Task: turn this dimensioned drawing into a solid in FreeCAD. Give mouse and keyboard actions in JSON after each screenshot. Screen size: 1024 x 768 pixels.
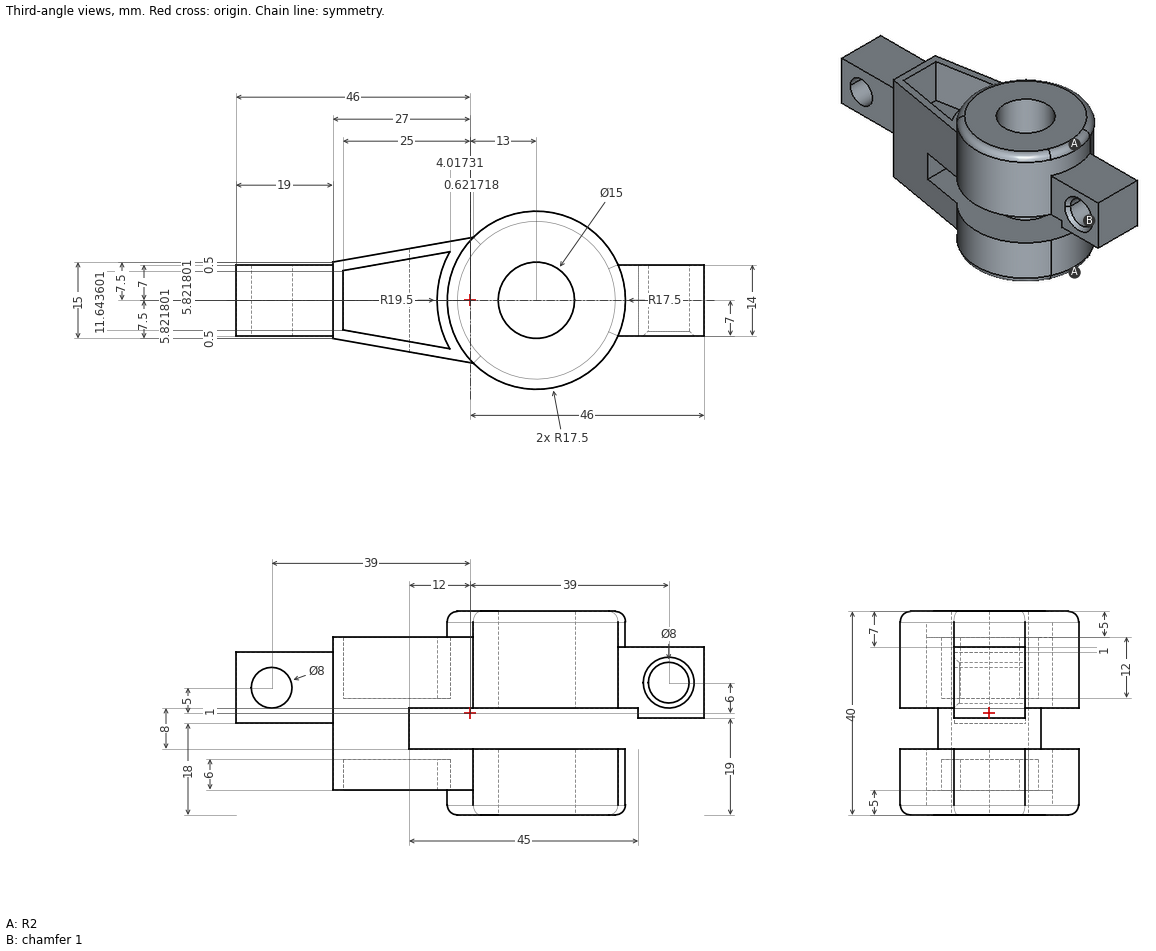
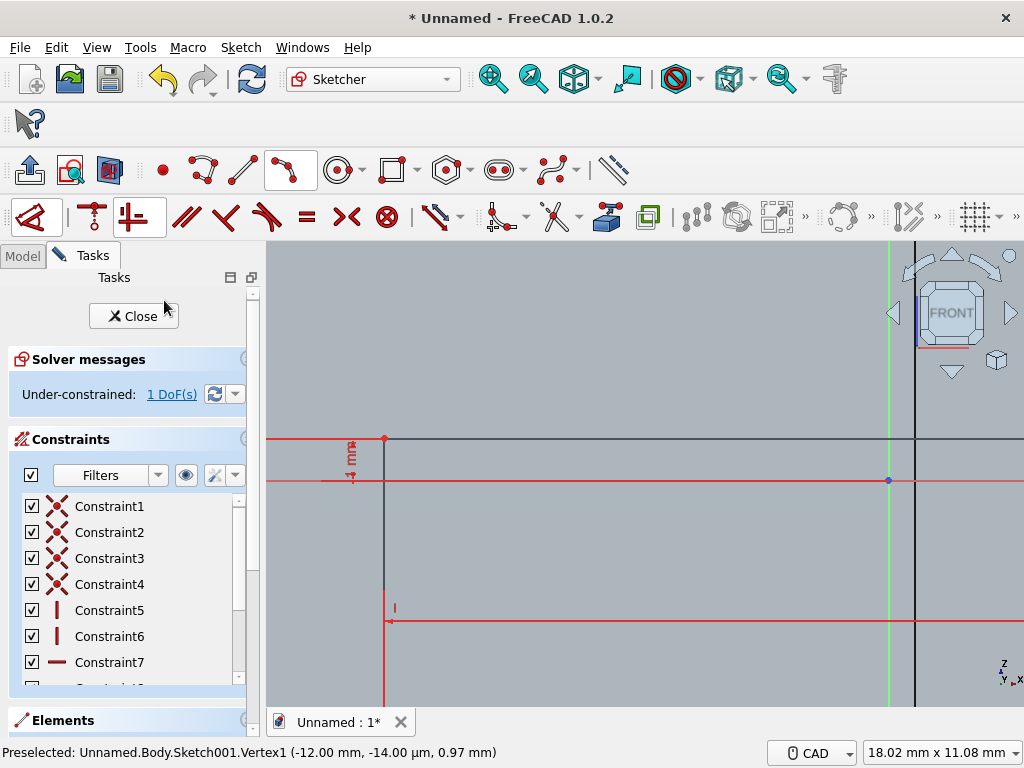
{"action": "scroll", "coordinate": [386, 440], "scroll_direction": "down", "scroll_amount": 8}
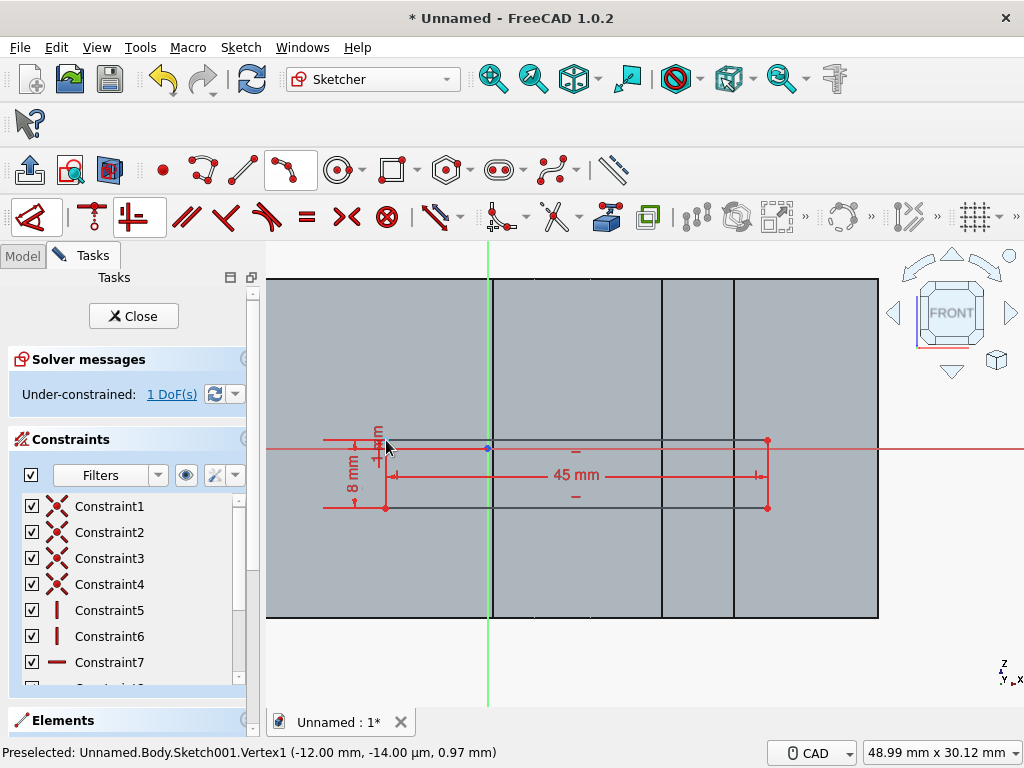
{"action": "left_click", "coordinate": [386, 440]}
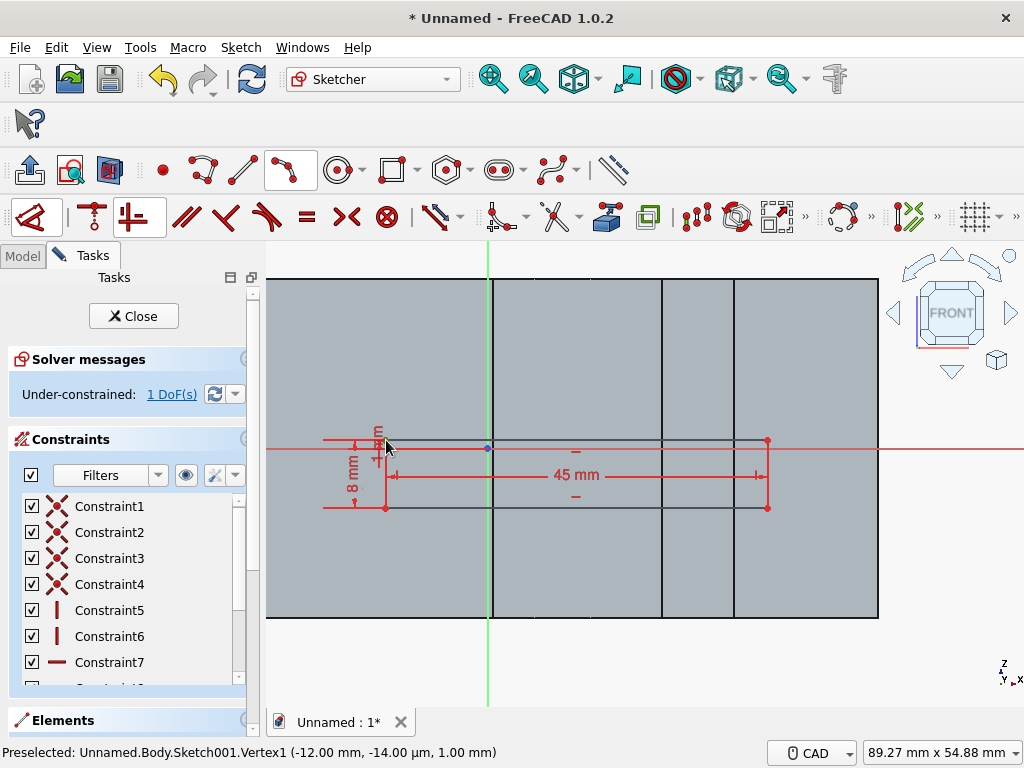
{"action": "key", "text": "l"}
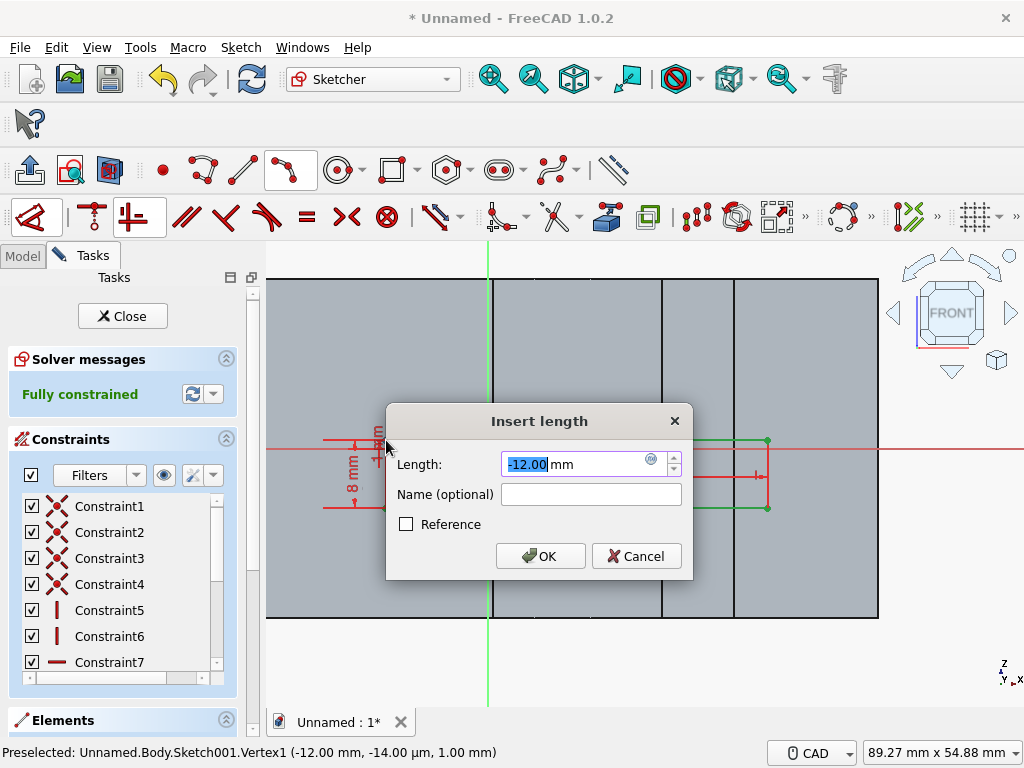
{"action": "type", "text": "-12"}
{"action": "key", "text": "Return"}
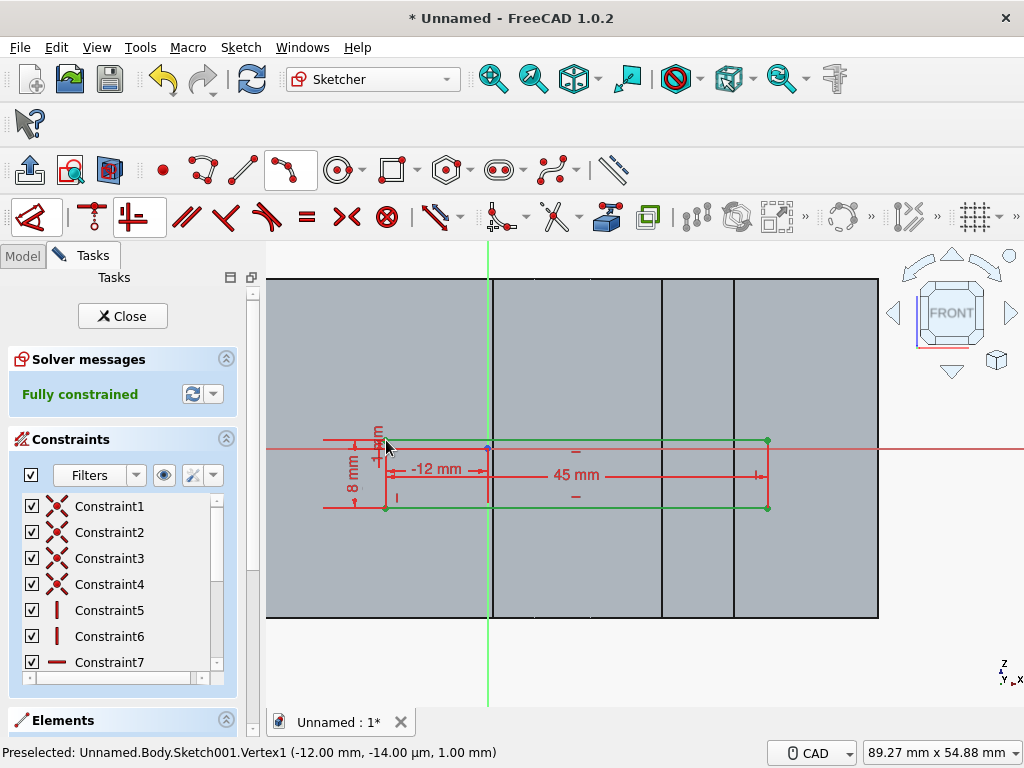
{"action": "left_click", "coordinate": [123, 316]}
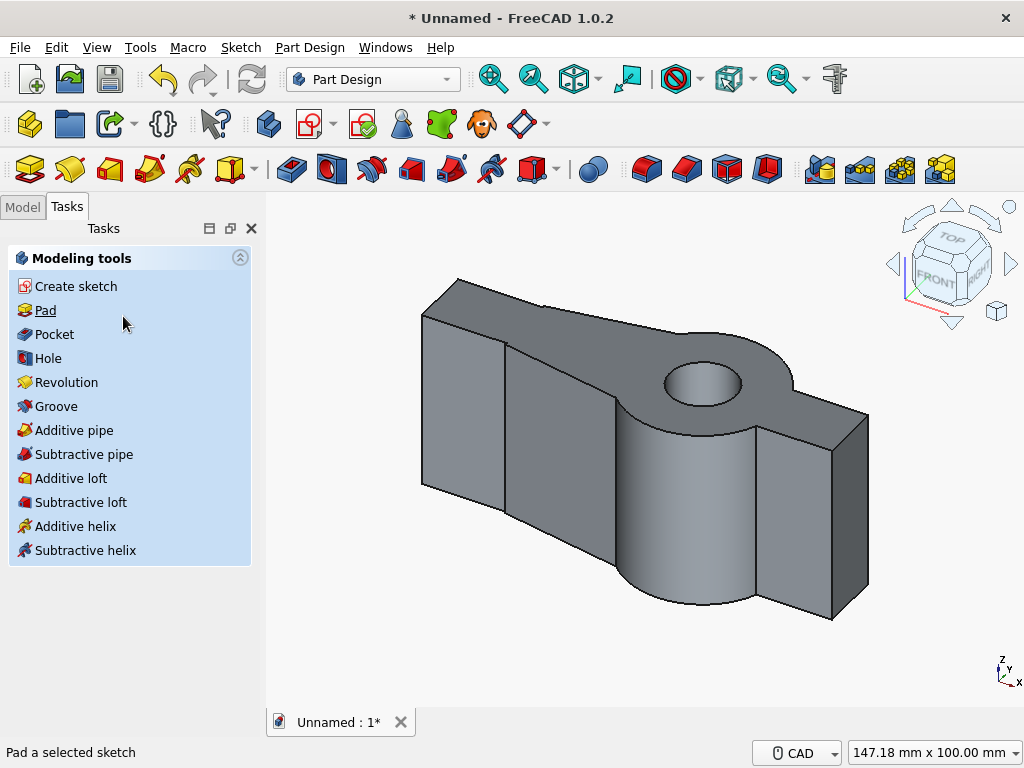
{"action": "left_click", "coordinate": [292, 170]}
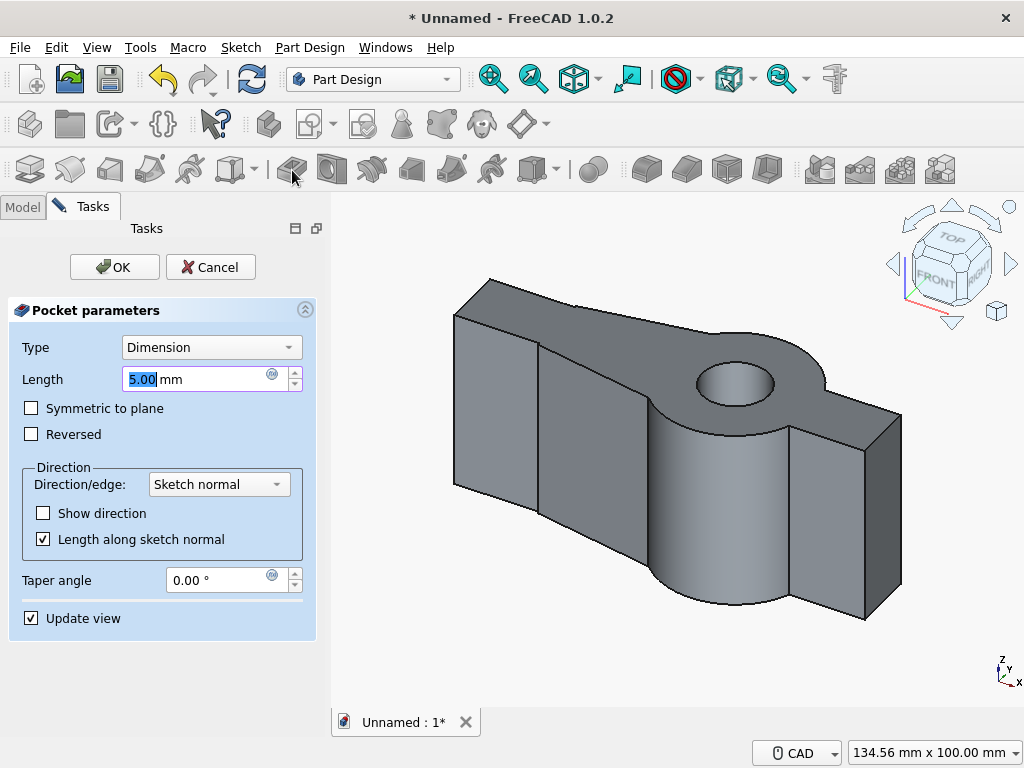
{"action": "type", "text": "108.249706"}
{"action": "key", "text": "Tab"}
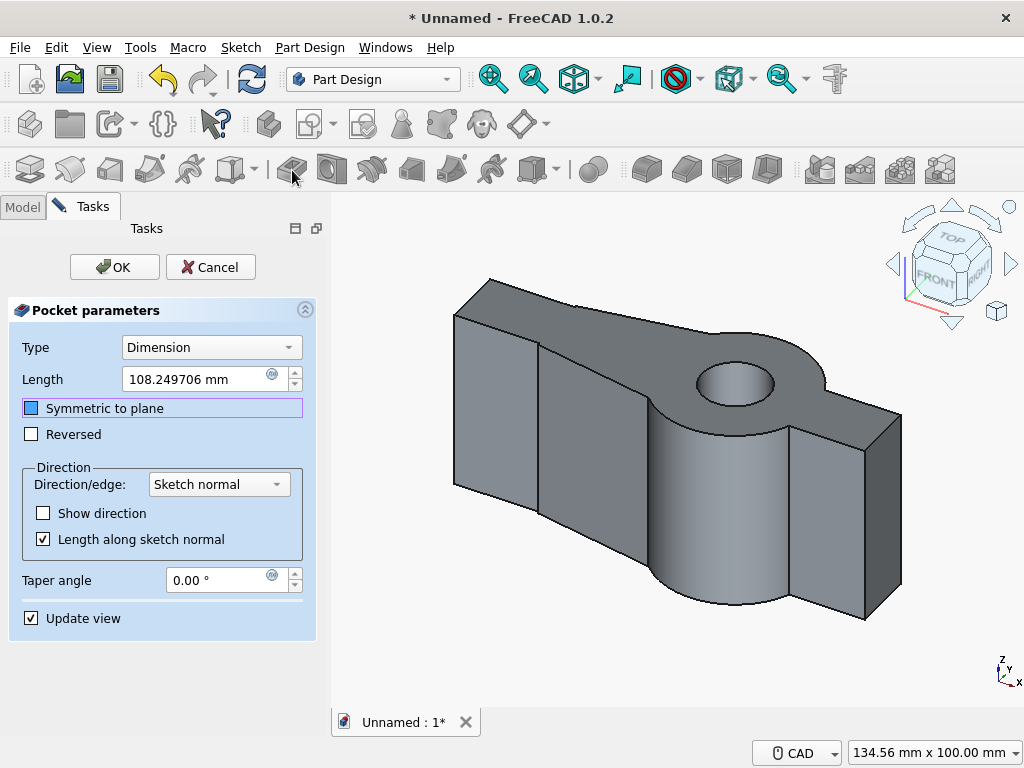
{"action": "left_click", "coordinate": [30, 408]}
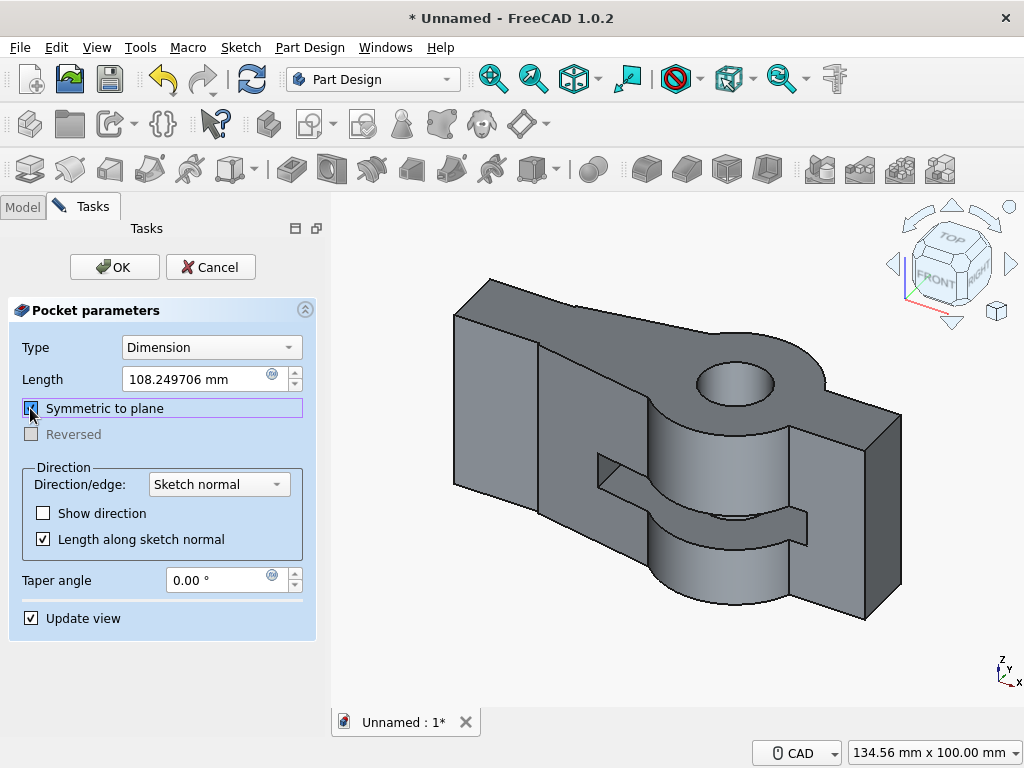
{"action": "left_click", "coordinate": [115, 267]}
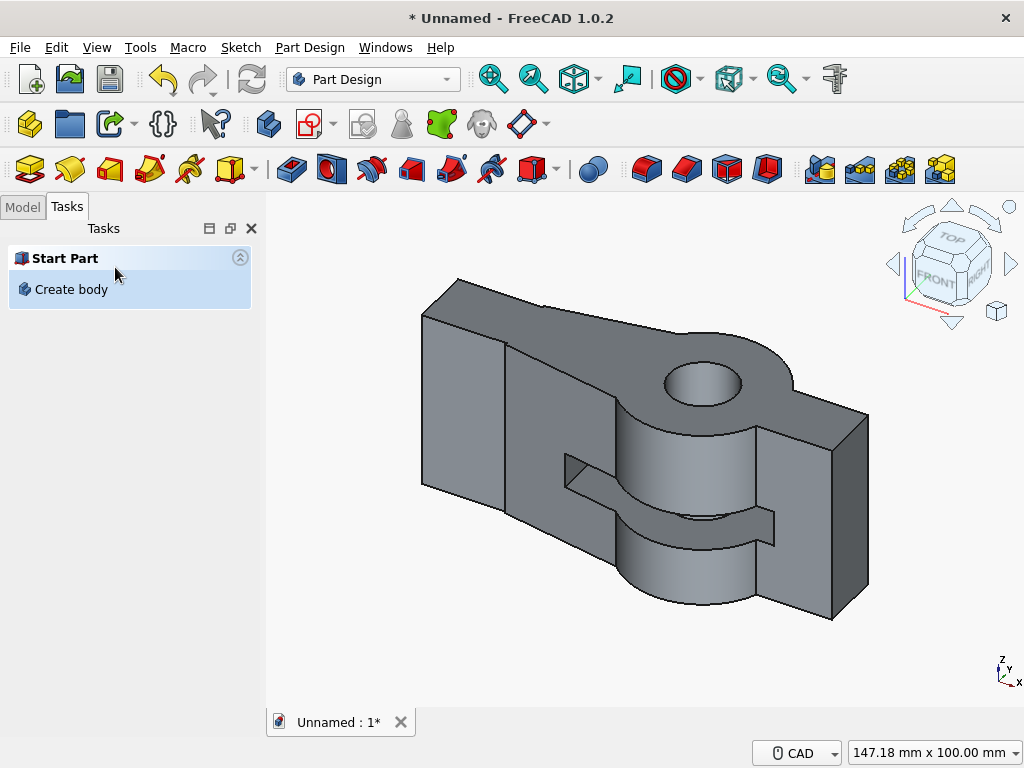
{"action": "left_click", "coordinate": [586, 345]}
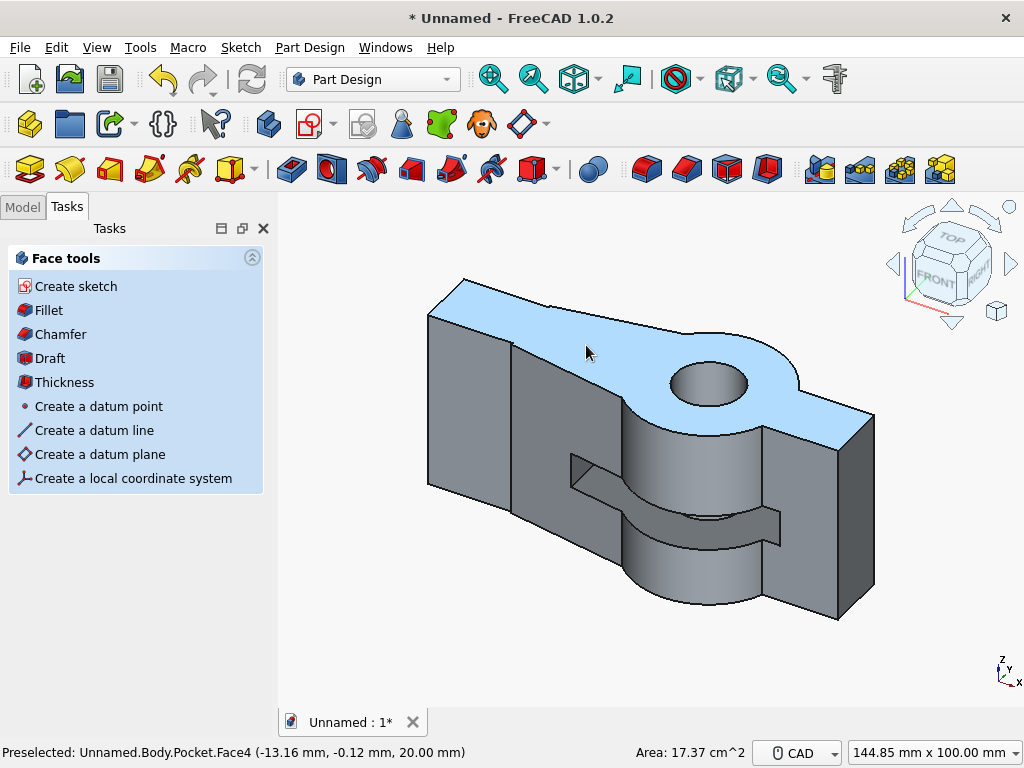
{"action": "left_click", "coordinate": [310, 124]}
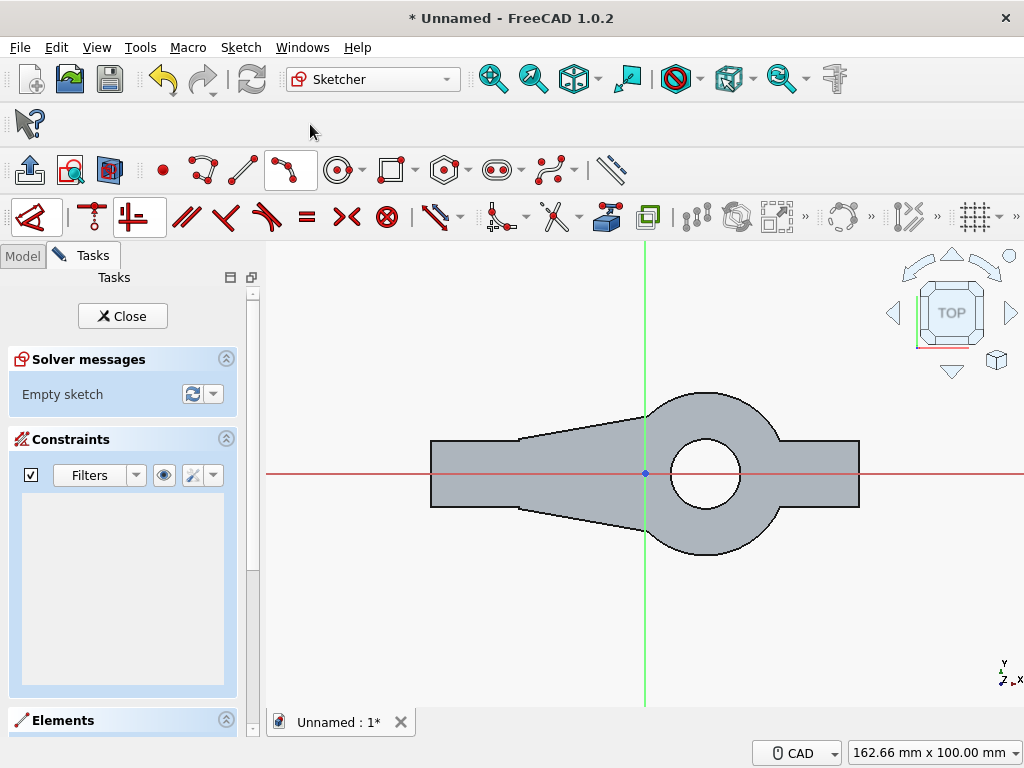
{"action": "scroll", "coordinate": [576, 474], "scroll_direction": "down", "scroll_amount": 5}